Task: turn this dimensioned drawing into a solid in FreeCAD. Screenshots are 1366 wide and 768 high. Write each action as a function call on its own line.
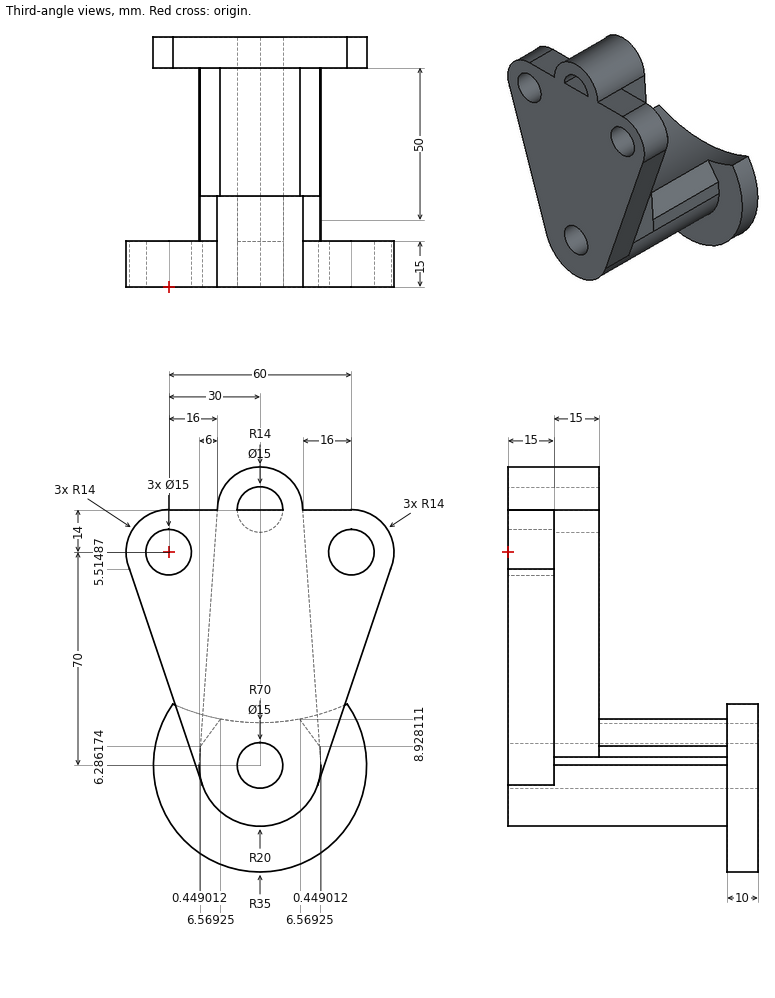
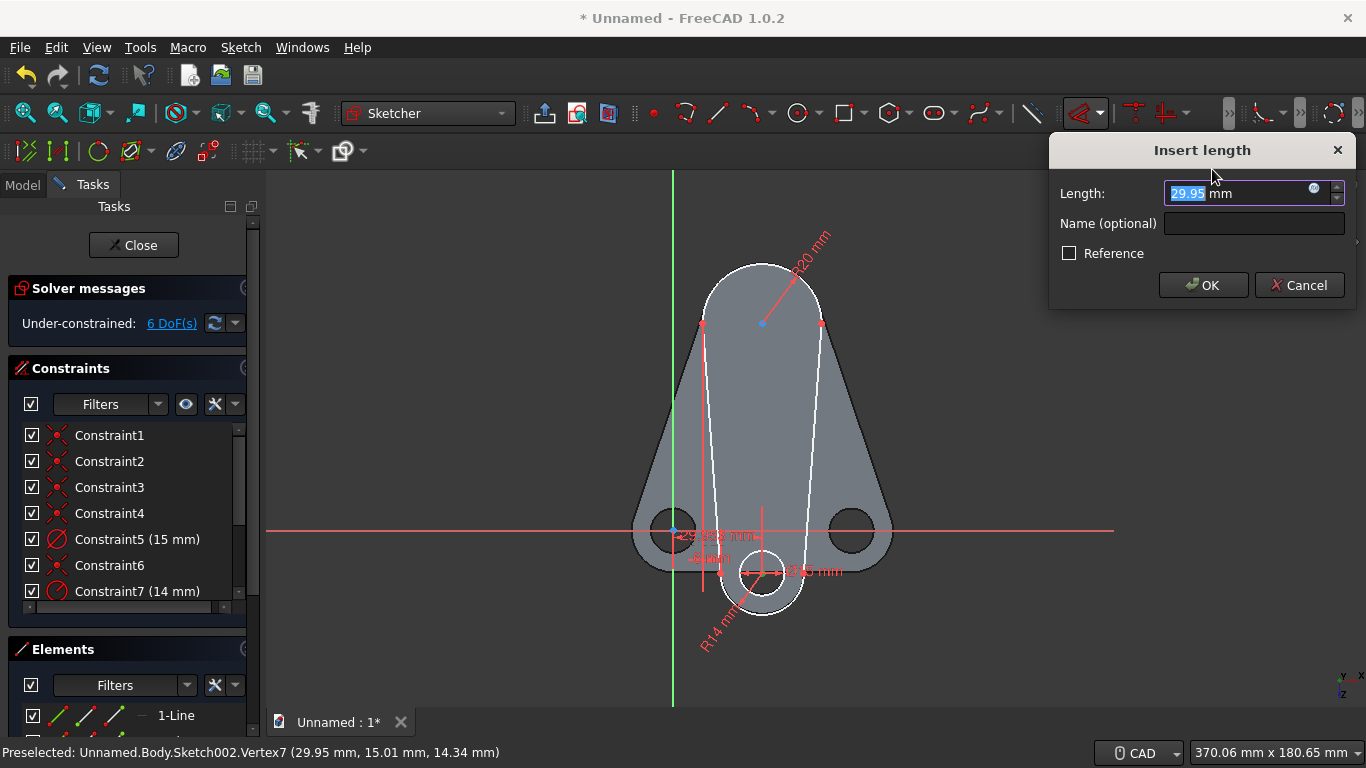
text(30)
key(Return)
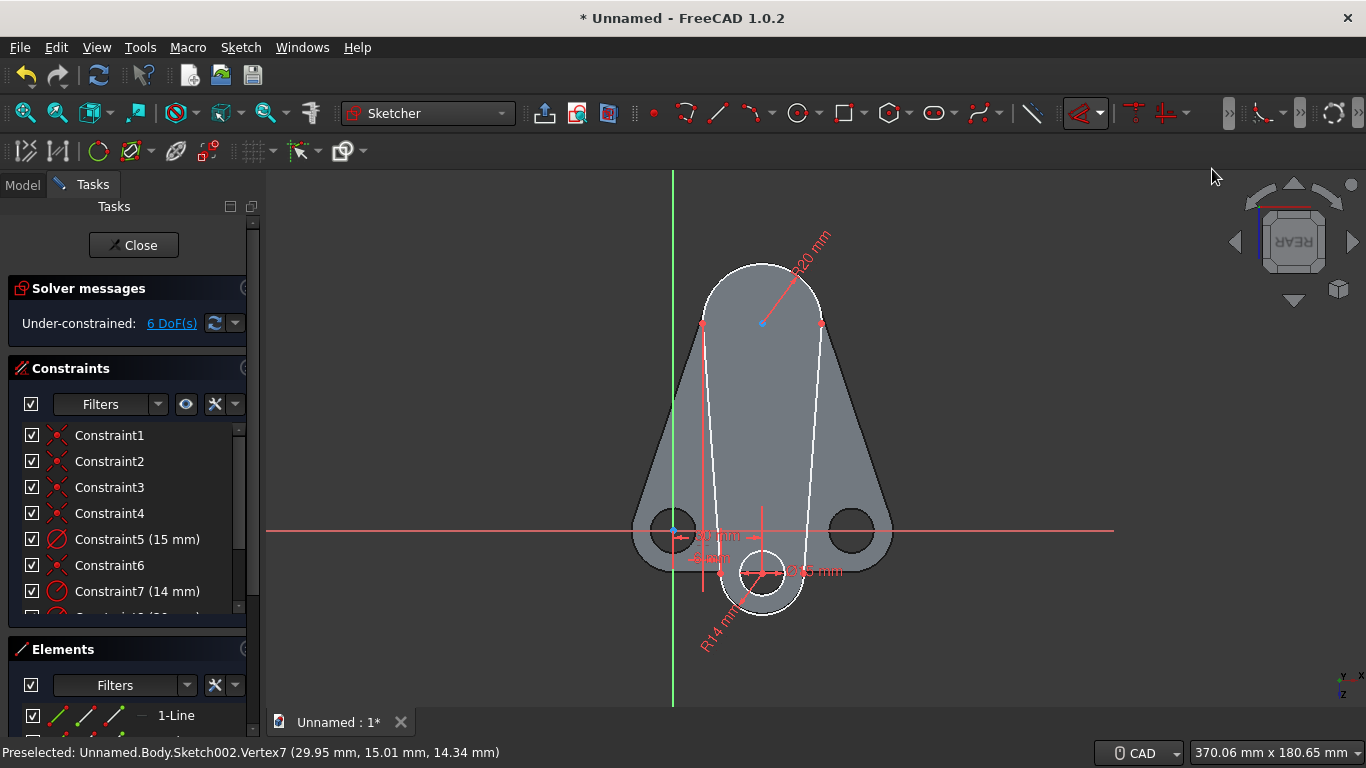
click(762, 573)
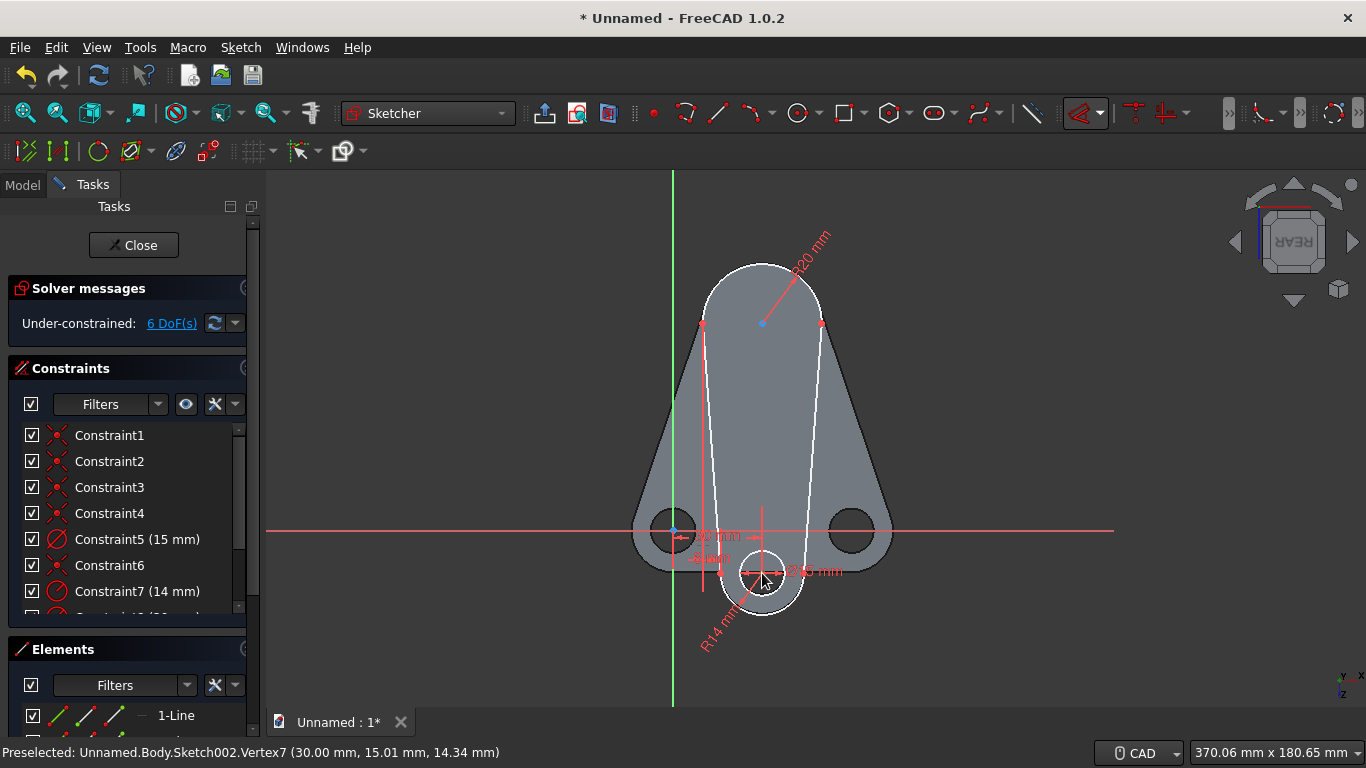
click(1102, 114)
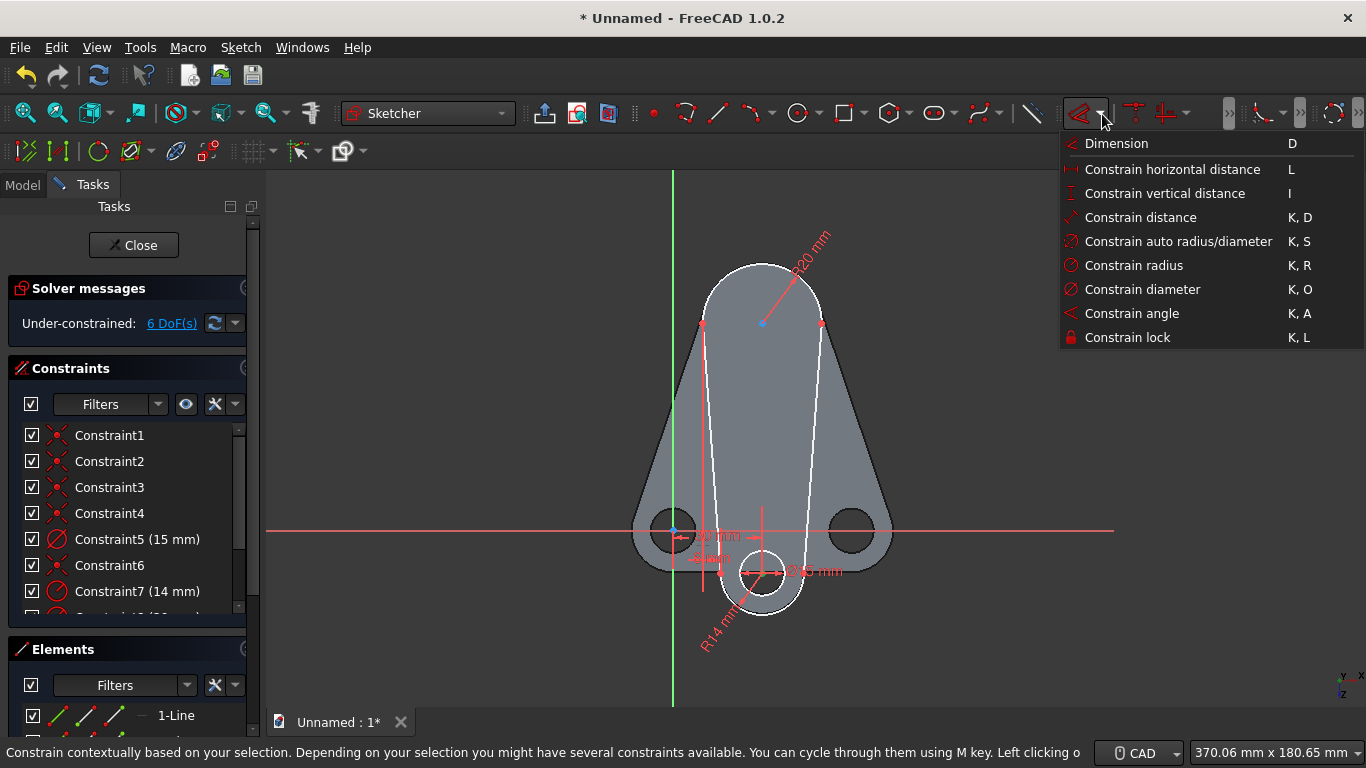
click(1212, 193)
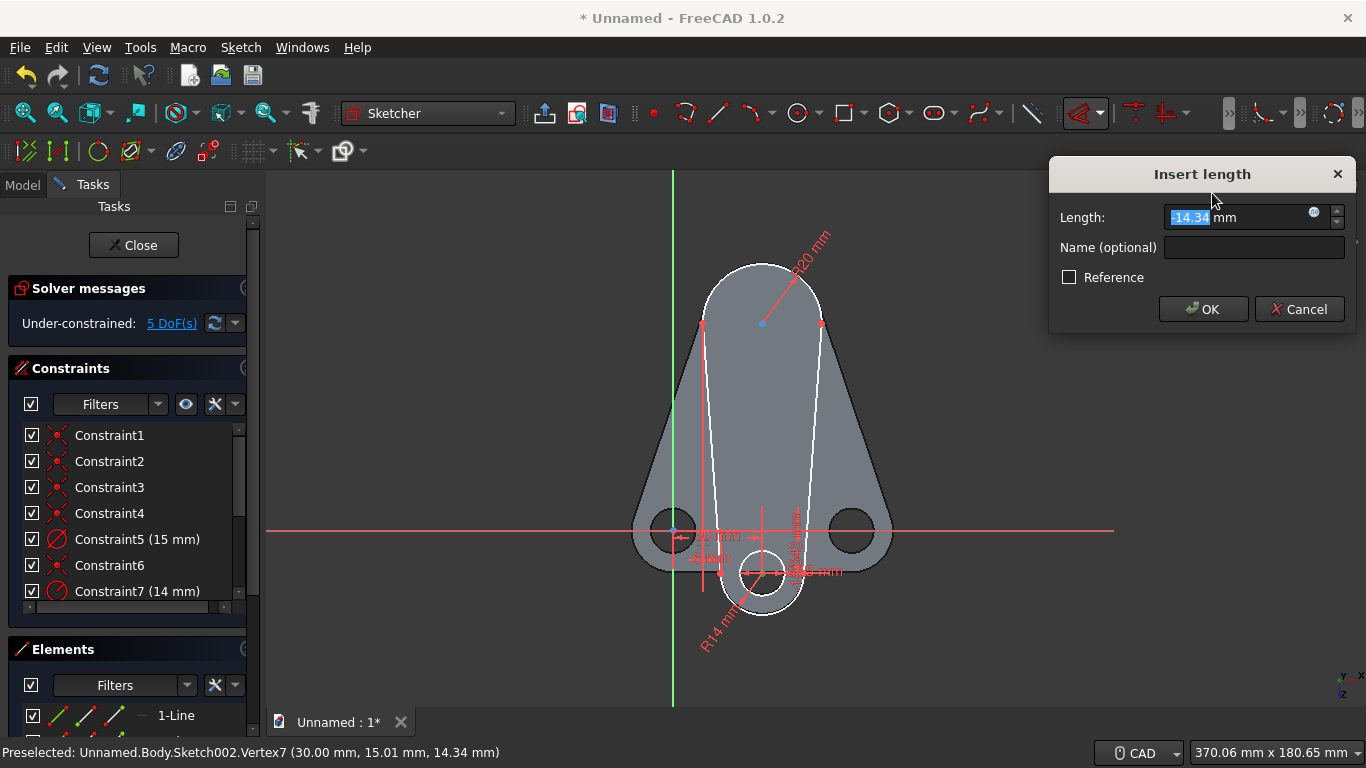
text(-14)
key(Return)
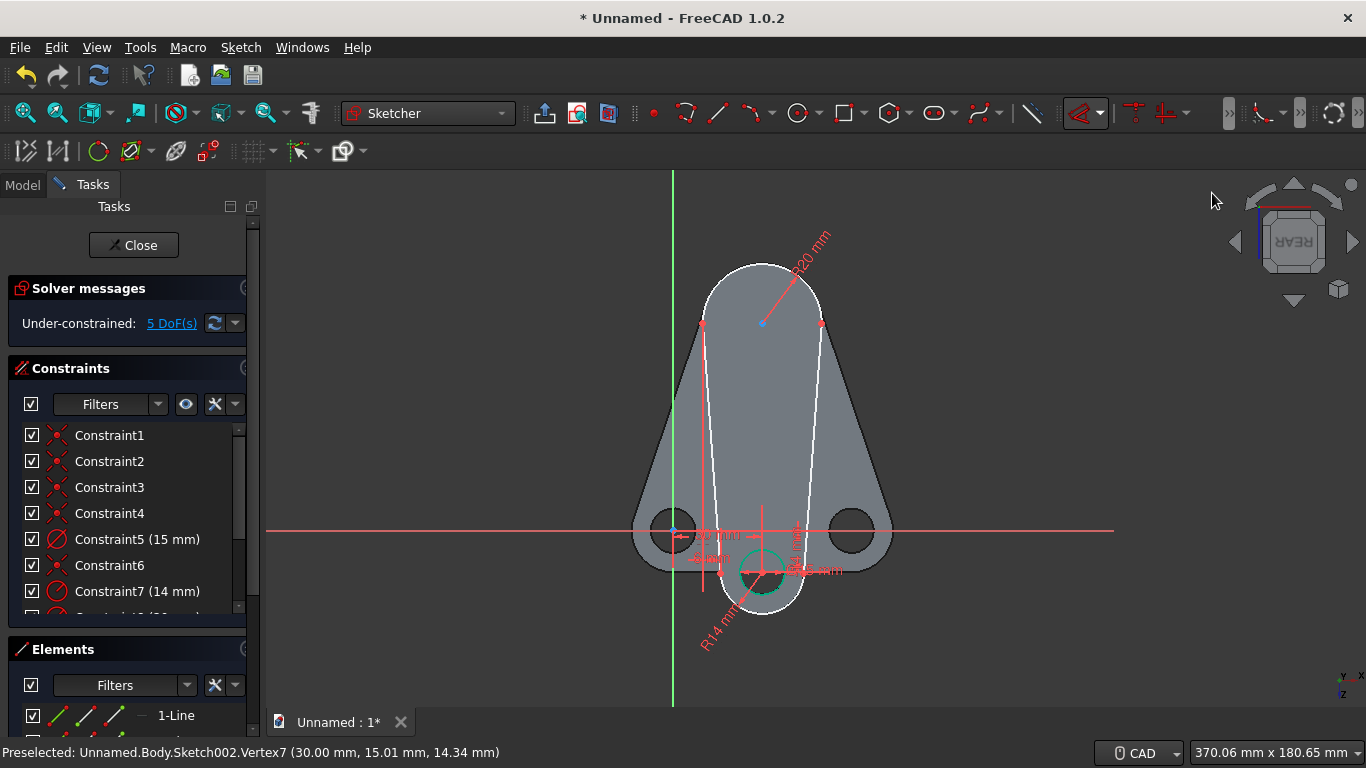
click(703, 324)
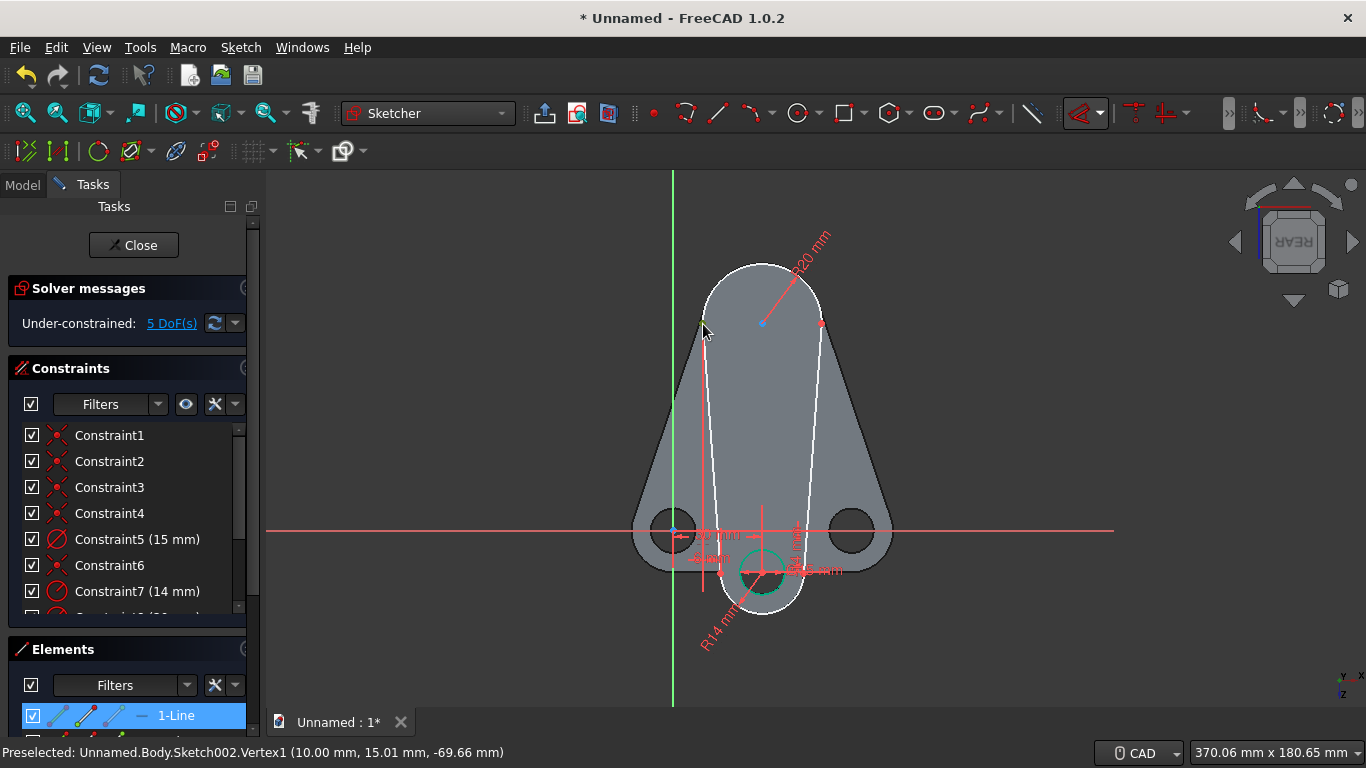
click(1102, 114)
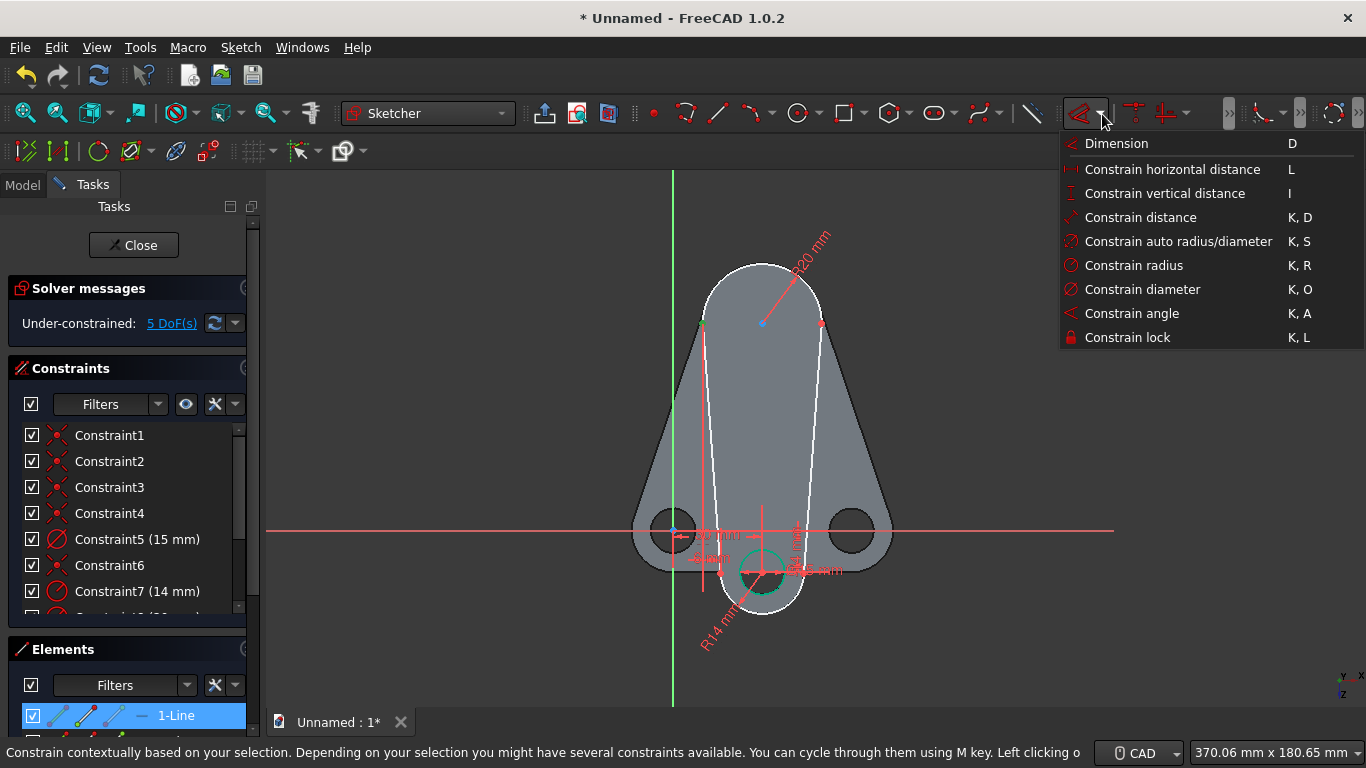
click(1212, 193)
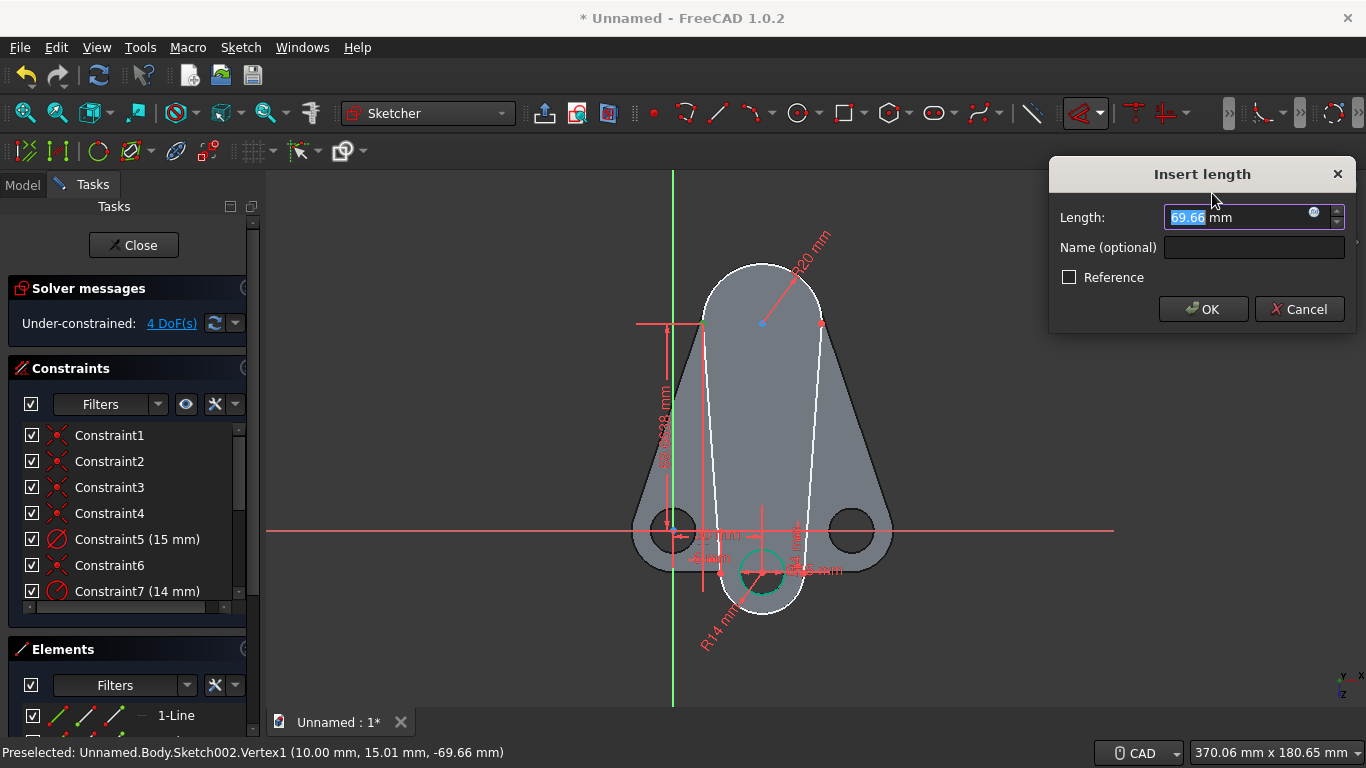
text(70)
key(Return)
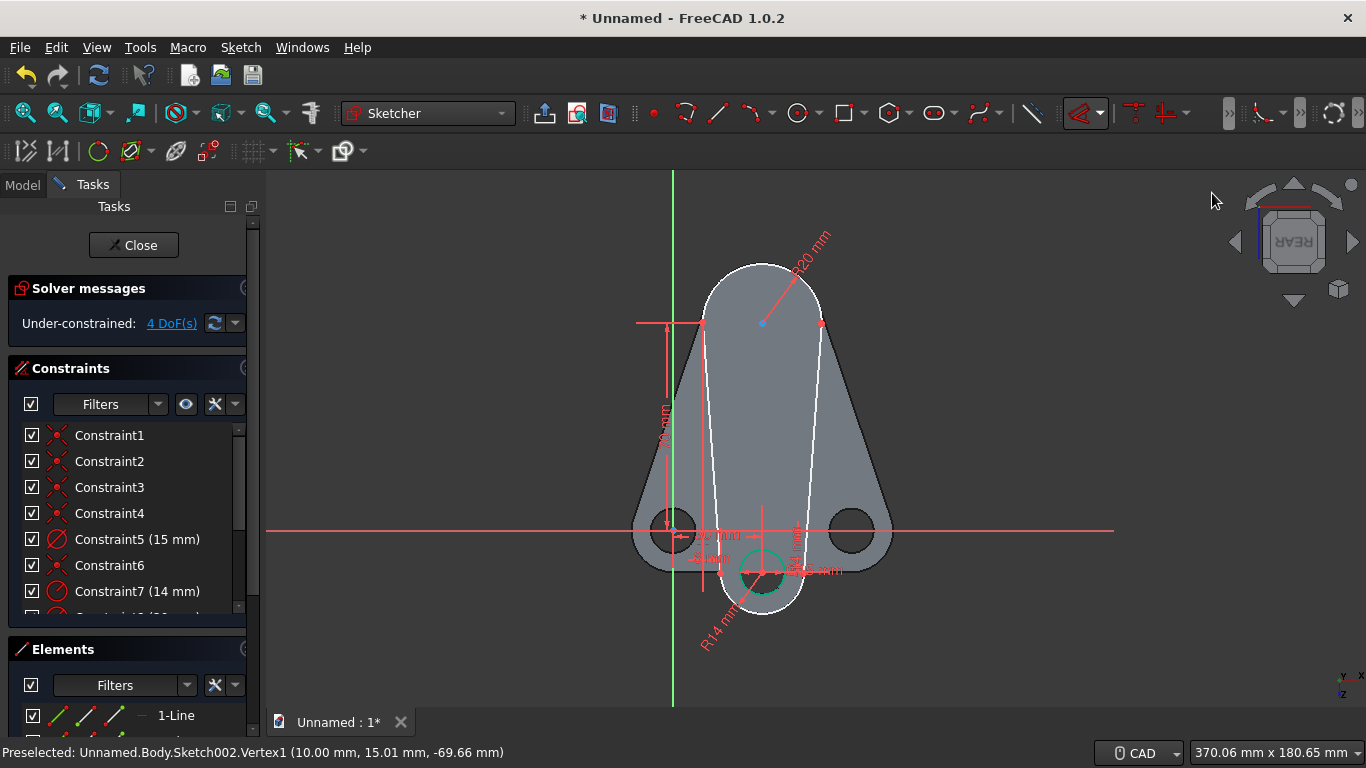
click(721, 573)